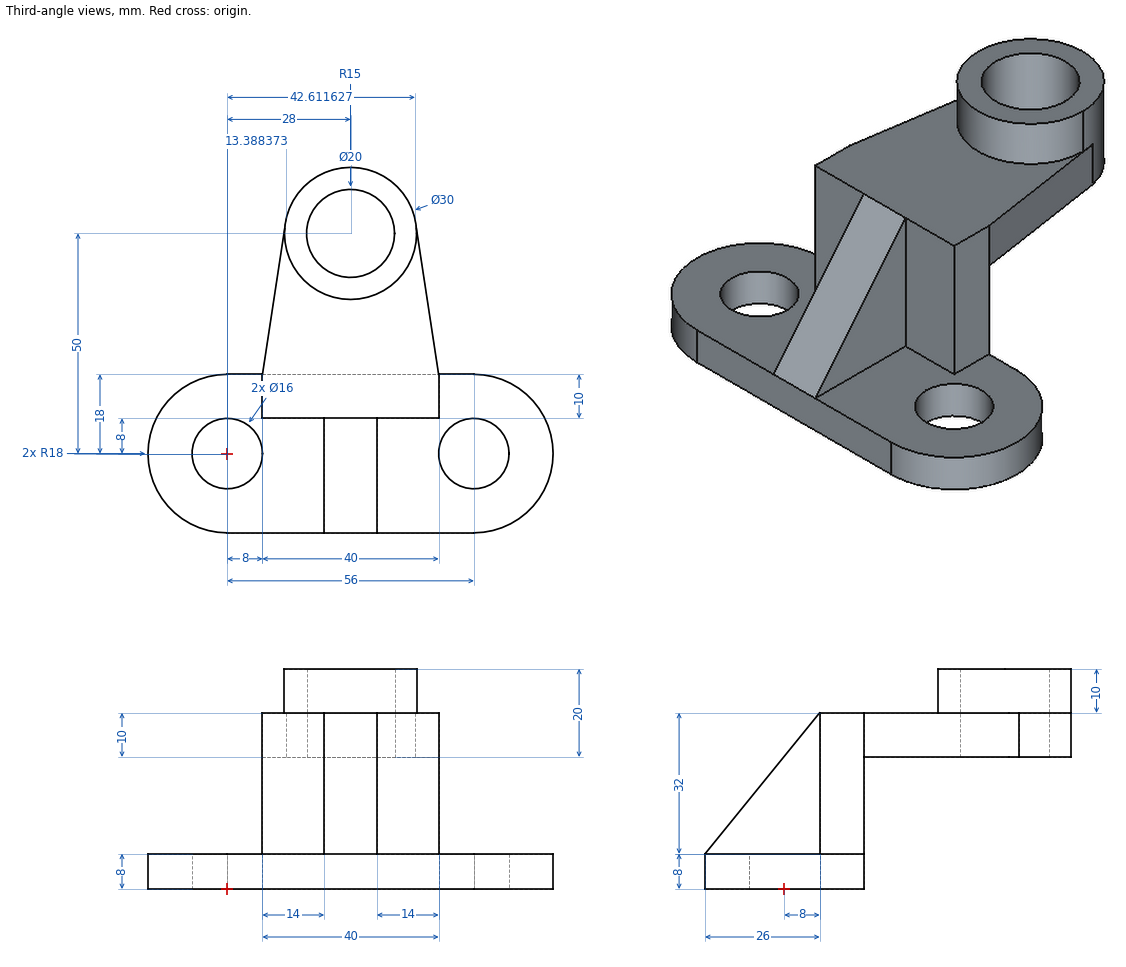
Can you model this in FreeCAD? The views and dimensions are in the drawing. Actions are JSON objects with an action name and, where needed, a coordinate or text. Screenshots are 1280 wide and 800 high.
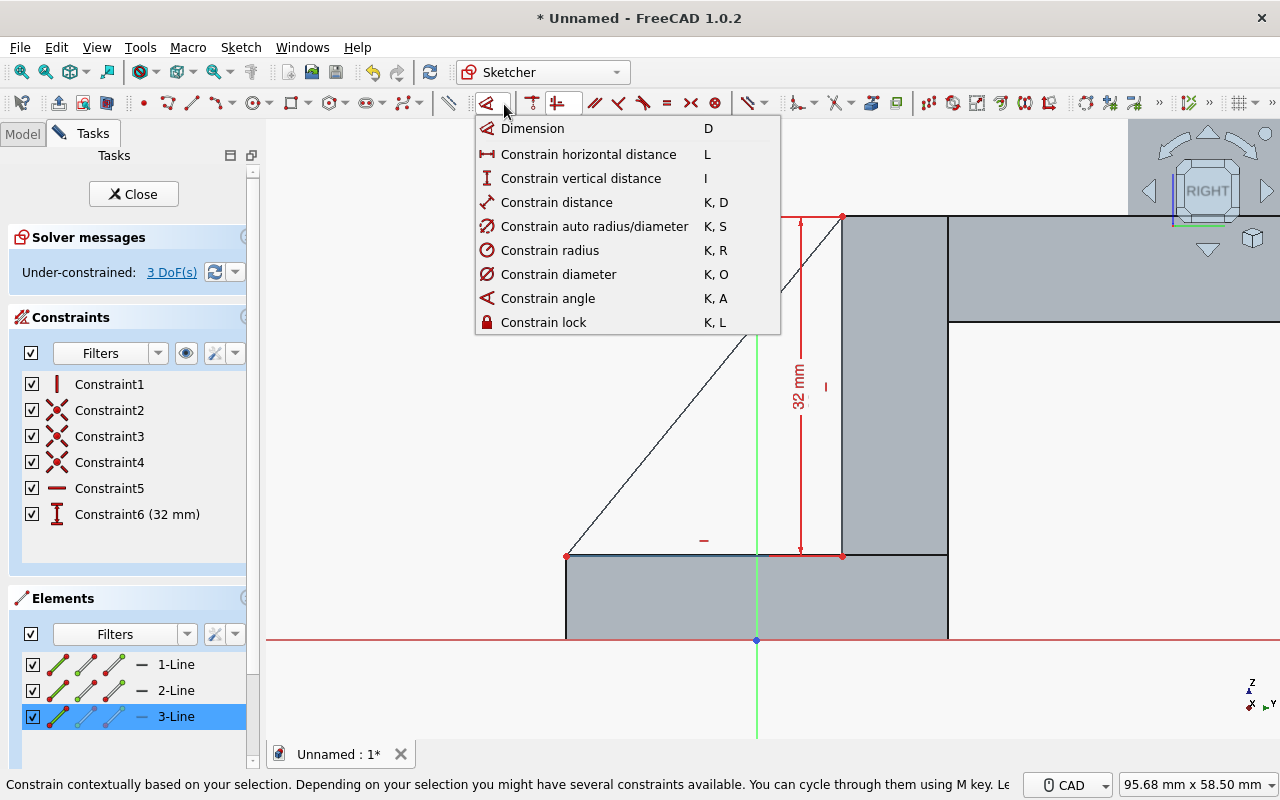
{"action": "left_click", "coordinate": [628, 154]}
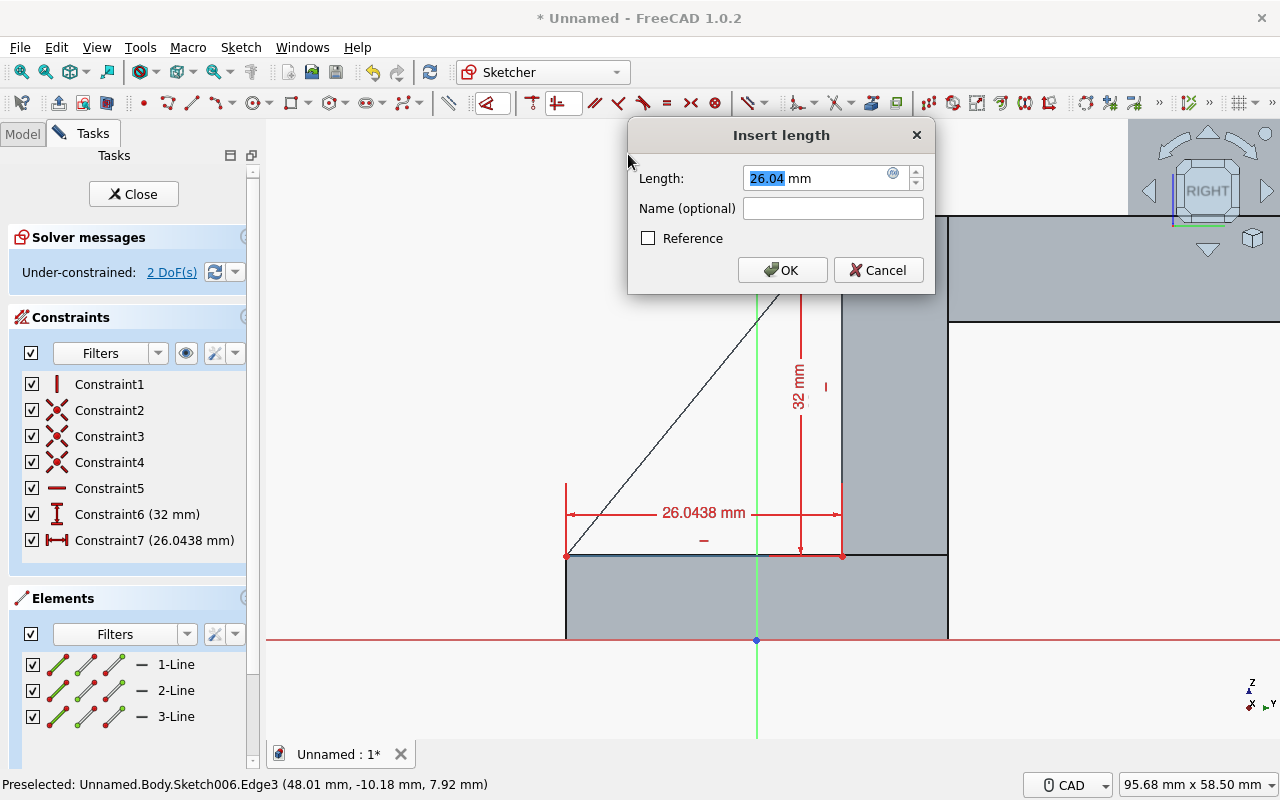
{"action": "type", "text": "26"}
{"action": "key", "text": "Return"}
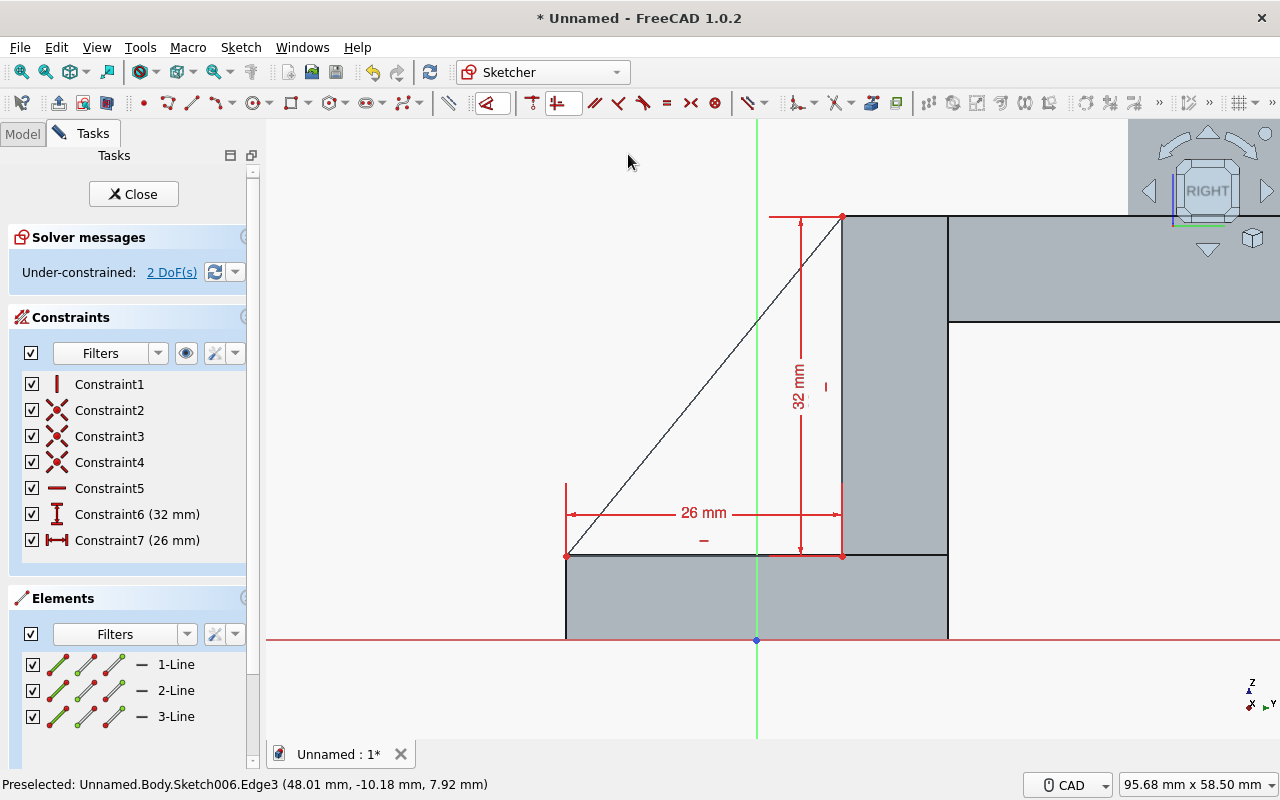
{"action": "left_click", "coordinate": [842, 556]}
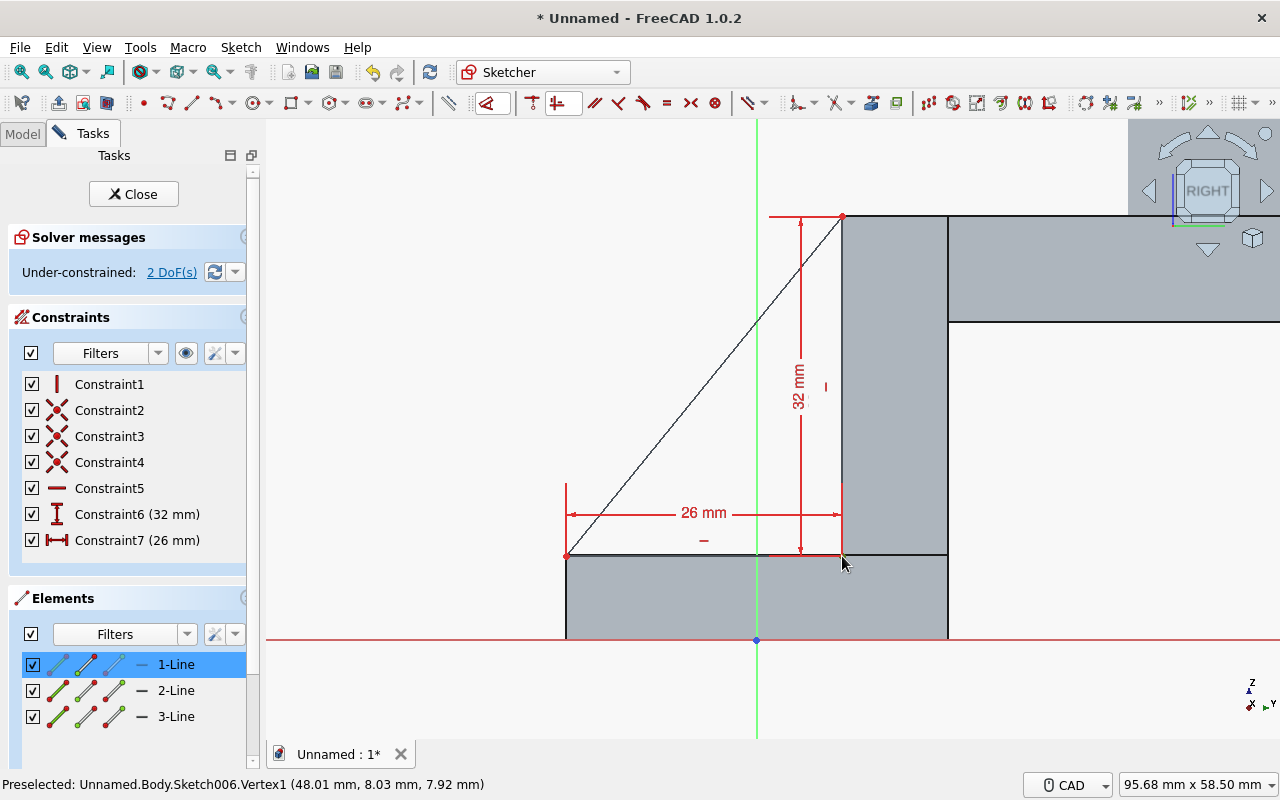
{"action": "key", "text": "l"}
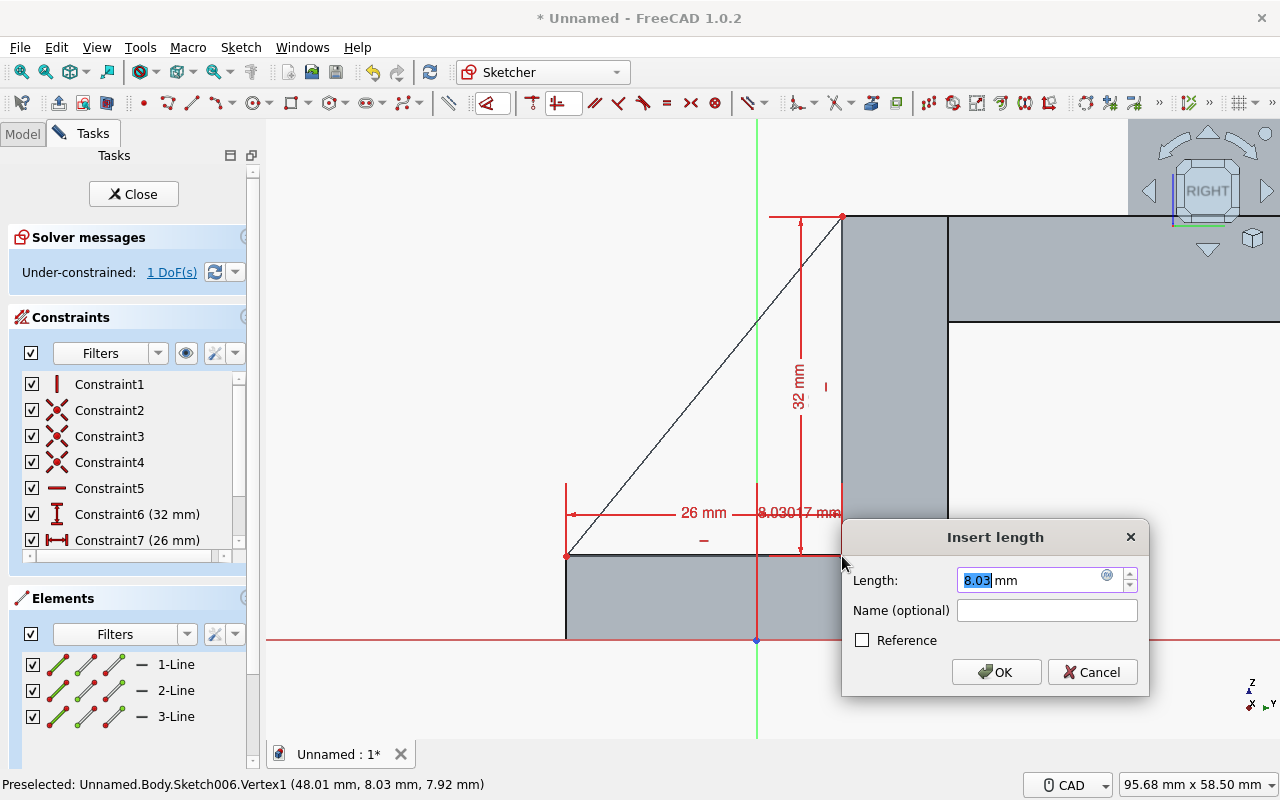
{"action": "type", "text": "8"}
{"action": "key", "text": "Return"}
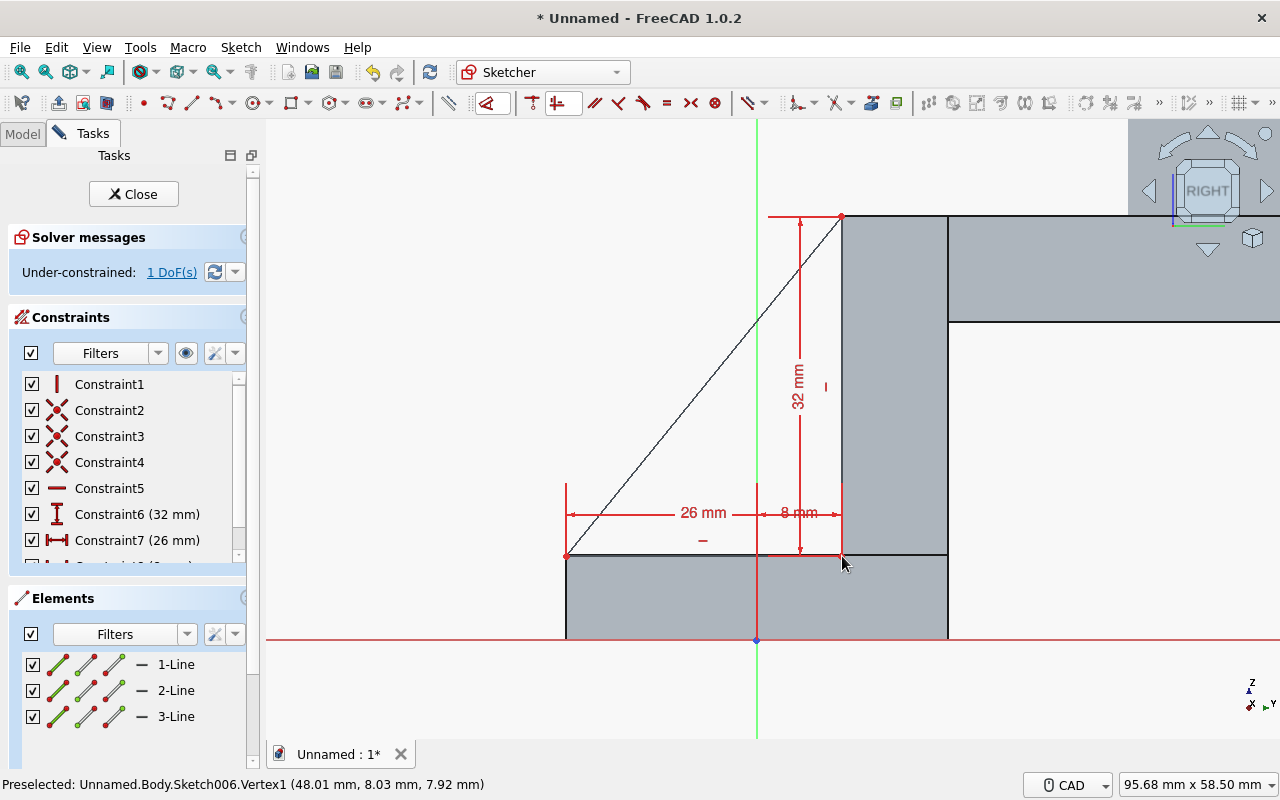
{"action": "left_click", "coordinate": [842, 556]}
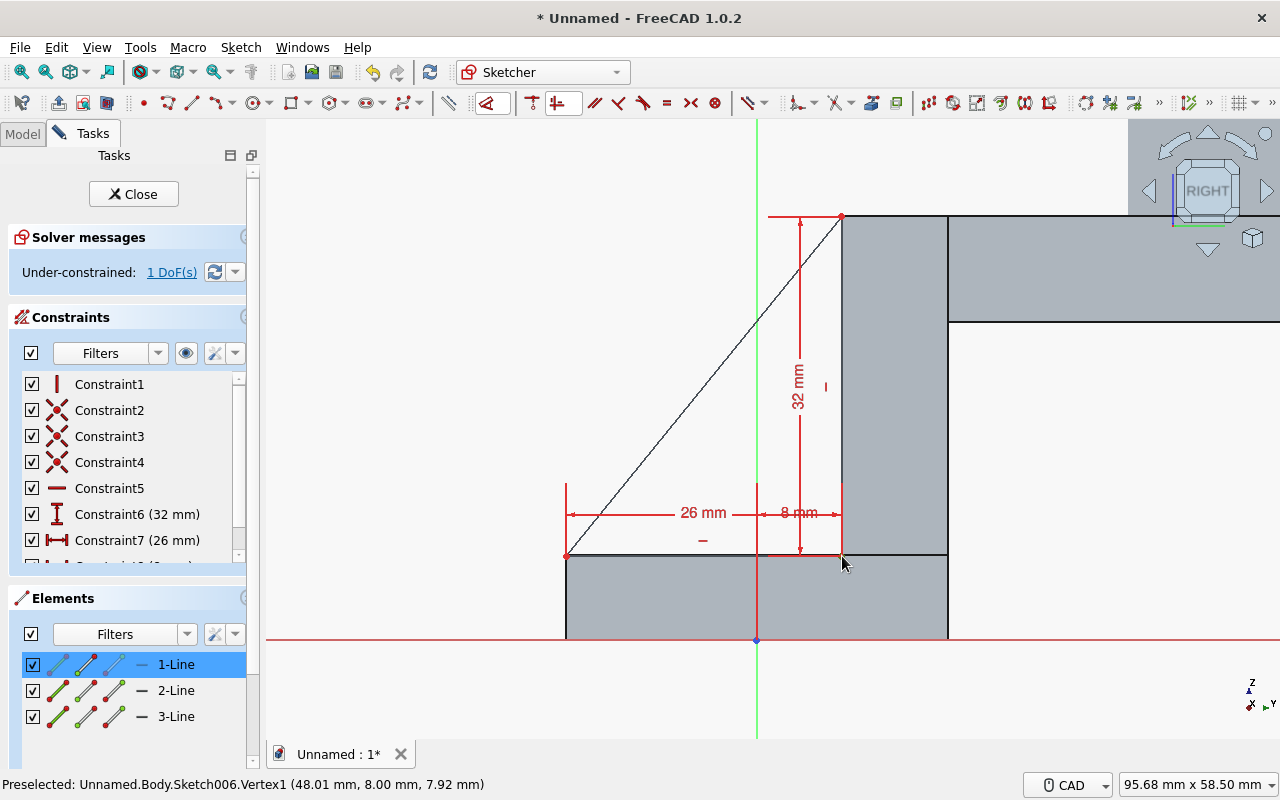
{"action": "left_click", "coordinate": [504, 104]}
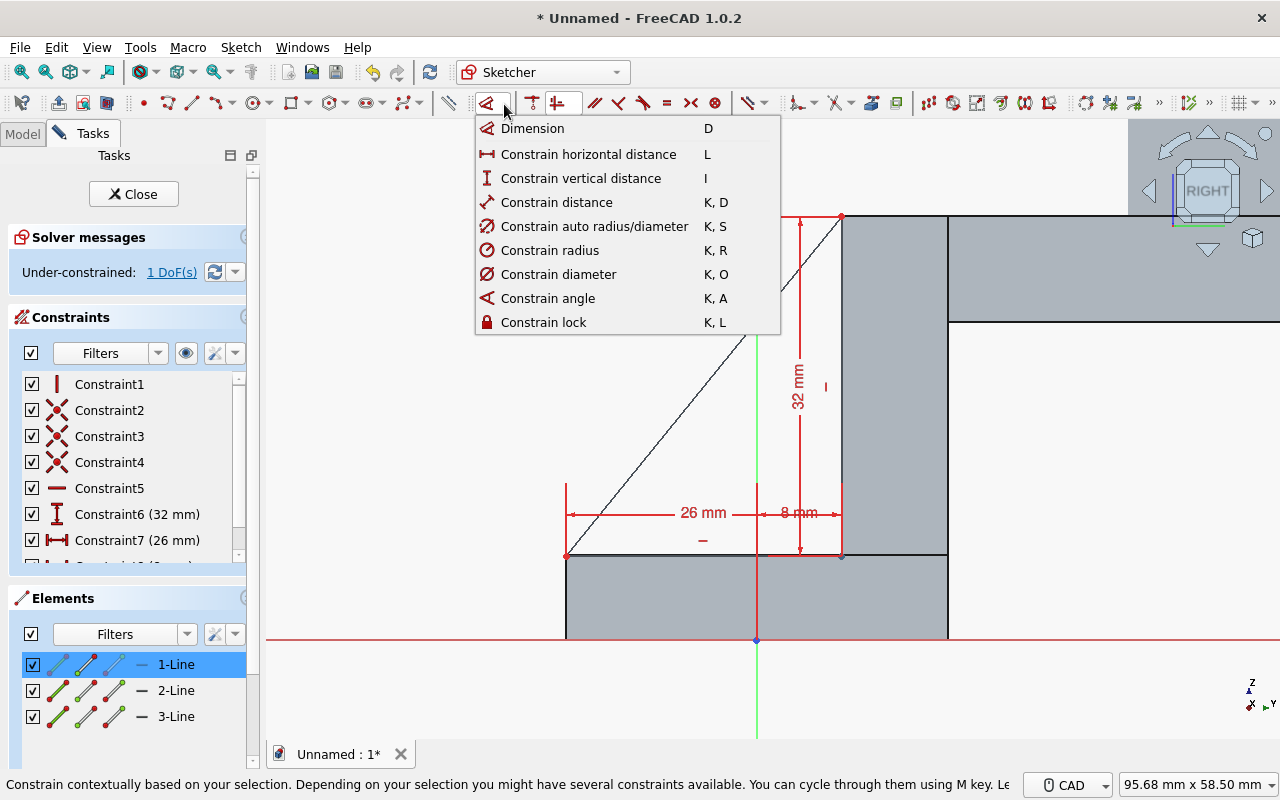
{"action": "left_click", "coordinate": [628, 178]}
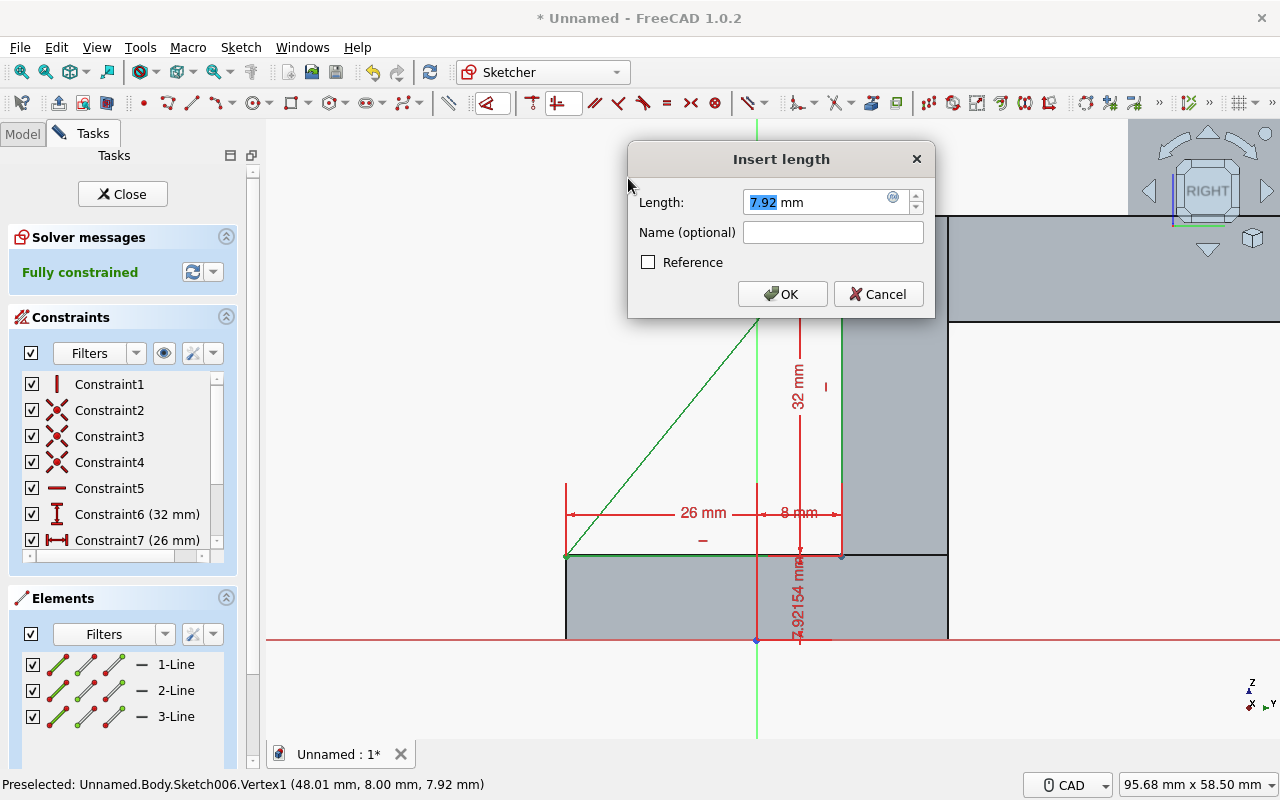
{"action": "type", "text": "8"}
{"action": "key", "text": "Return"}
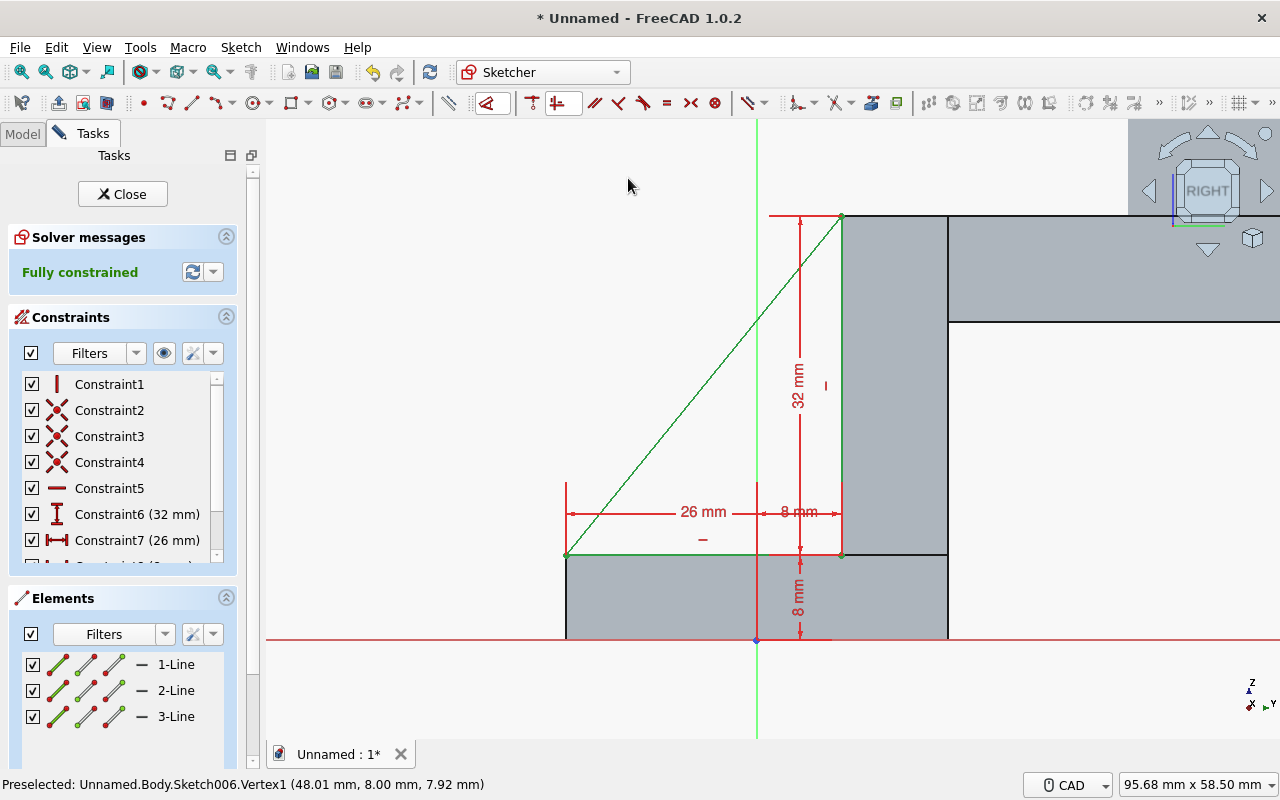
{"action": "left_click", "coordinate": [123, 194]}